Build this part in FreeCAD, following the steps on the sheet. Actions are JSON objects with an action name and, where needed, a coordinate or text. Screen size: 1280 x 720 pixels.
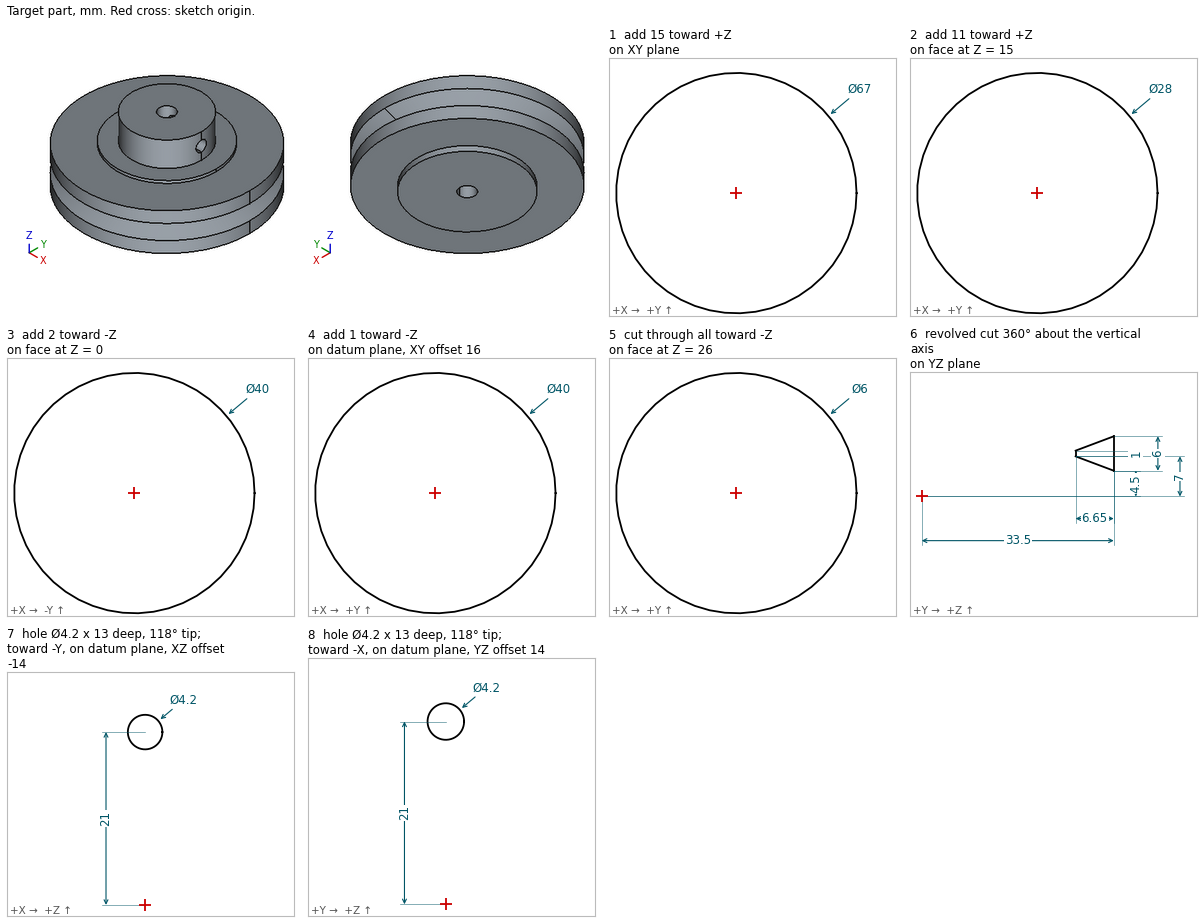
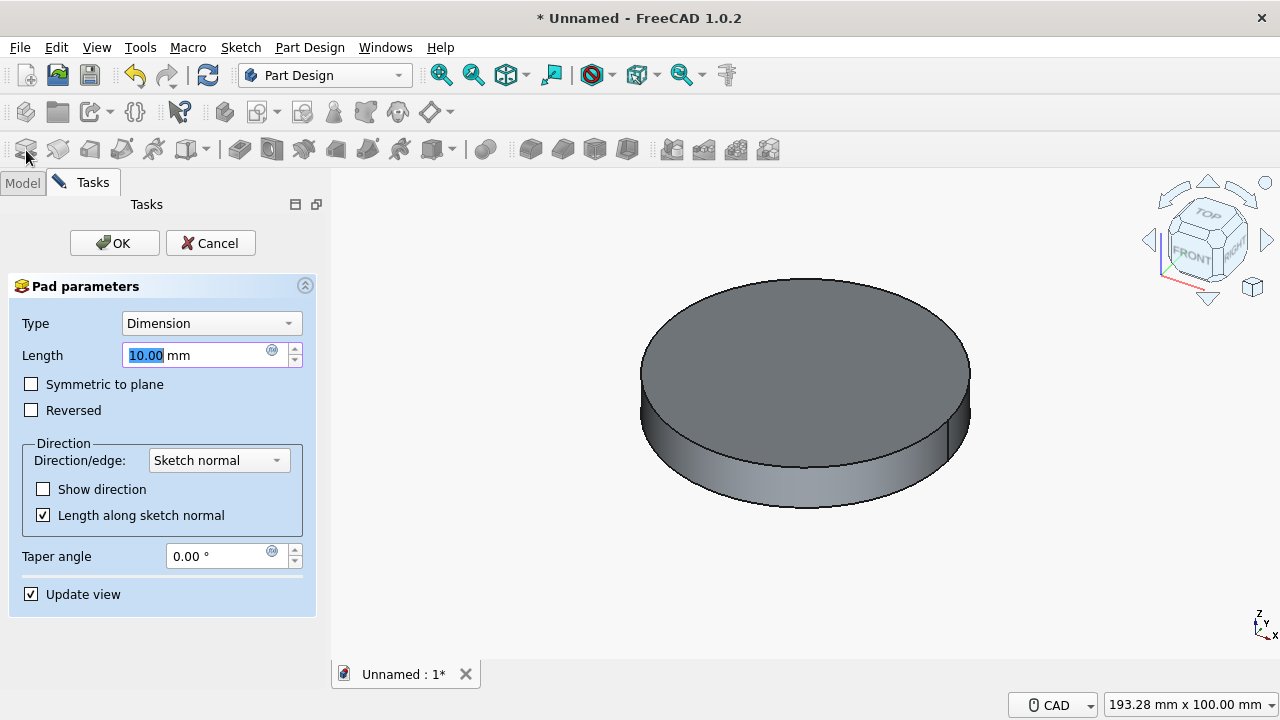
{"action": "type", "text": "15"}
{"action": "key", "text": "Tab"}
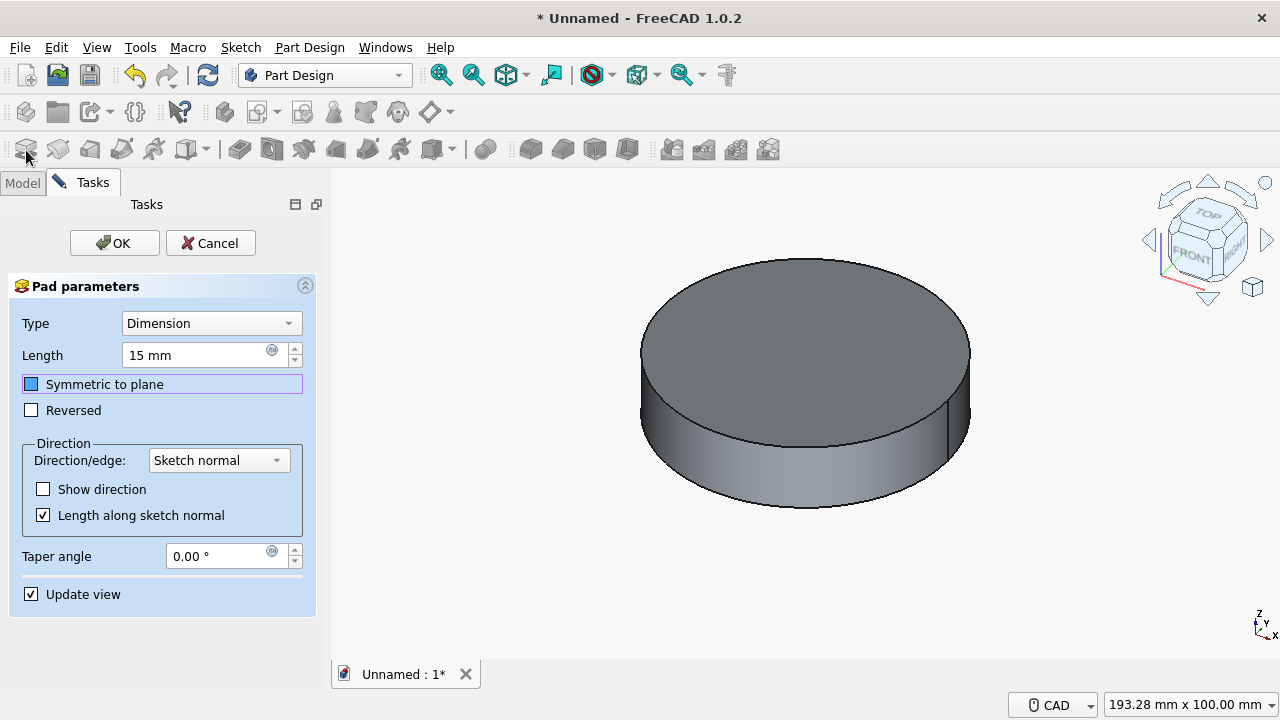
{"action": "left_click", "coordinate": [115, 243]}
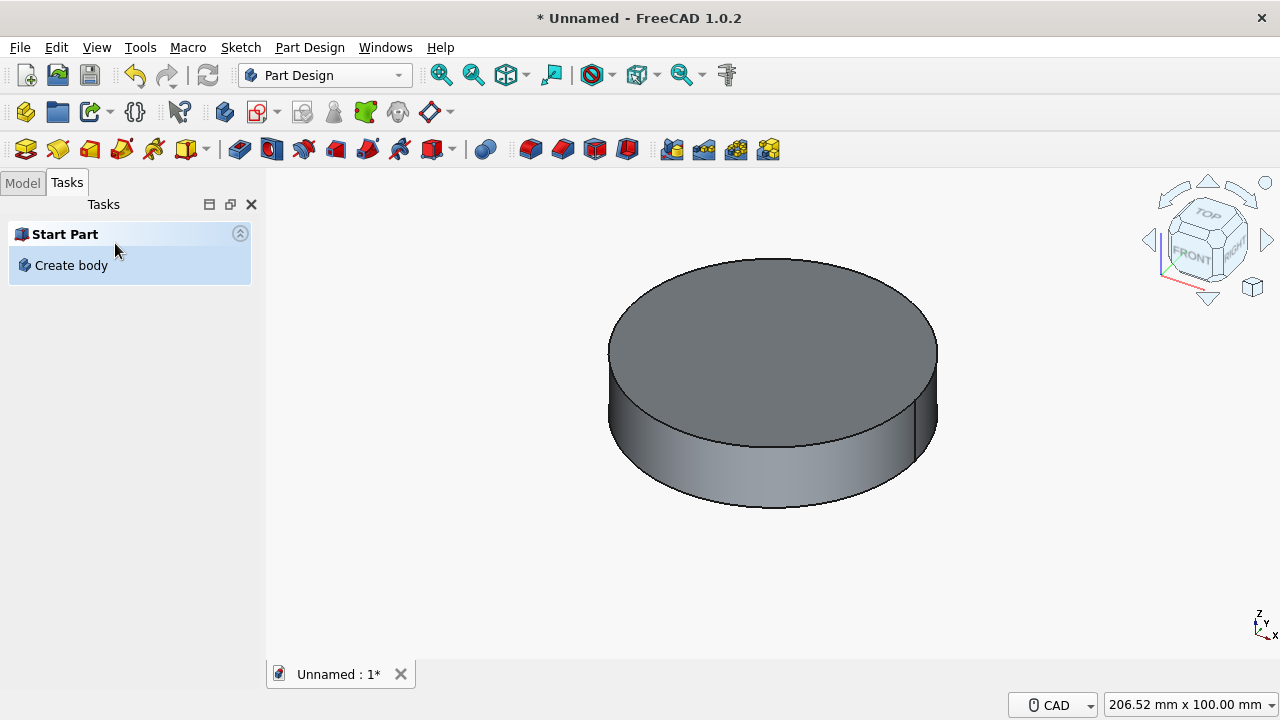
{"action": "left_click", "coordinate": [773, 352]}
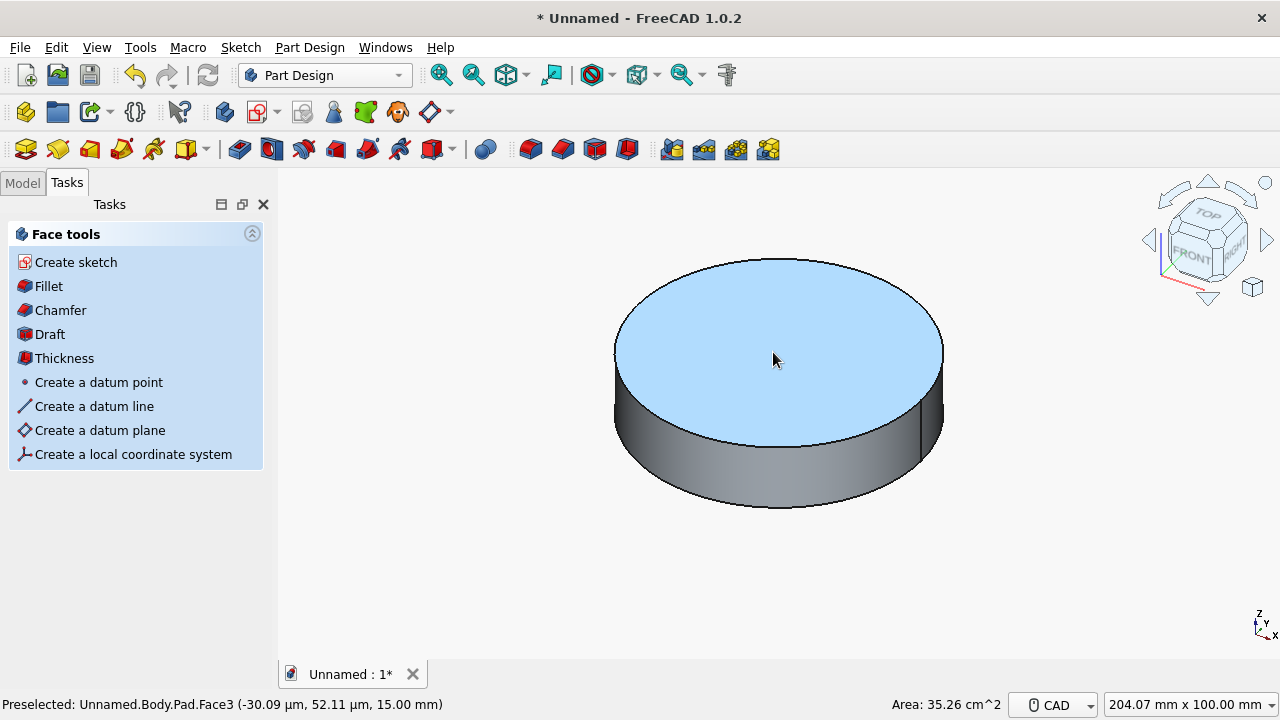
{"action": "left_click", "coordinate": [258, 112]}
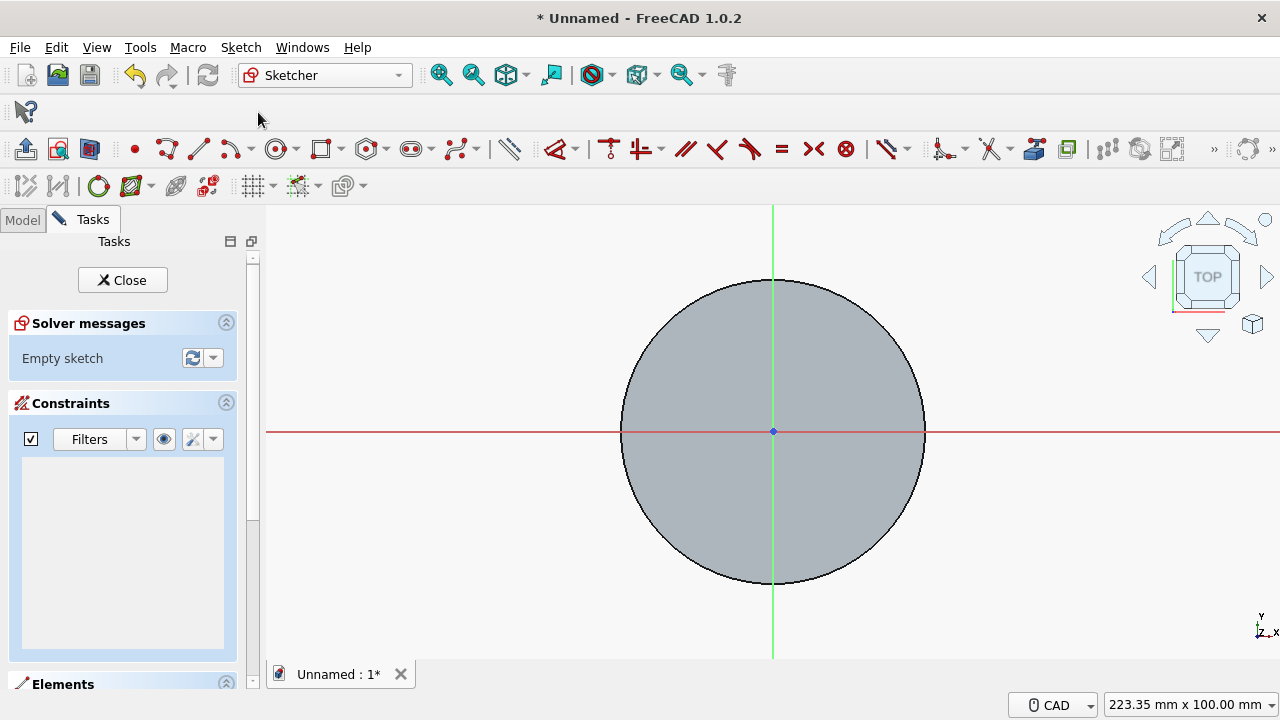
{"action": "scroll", "coordinate": [829, 432], "scroll_direction": "up", "scroll_amount": 4}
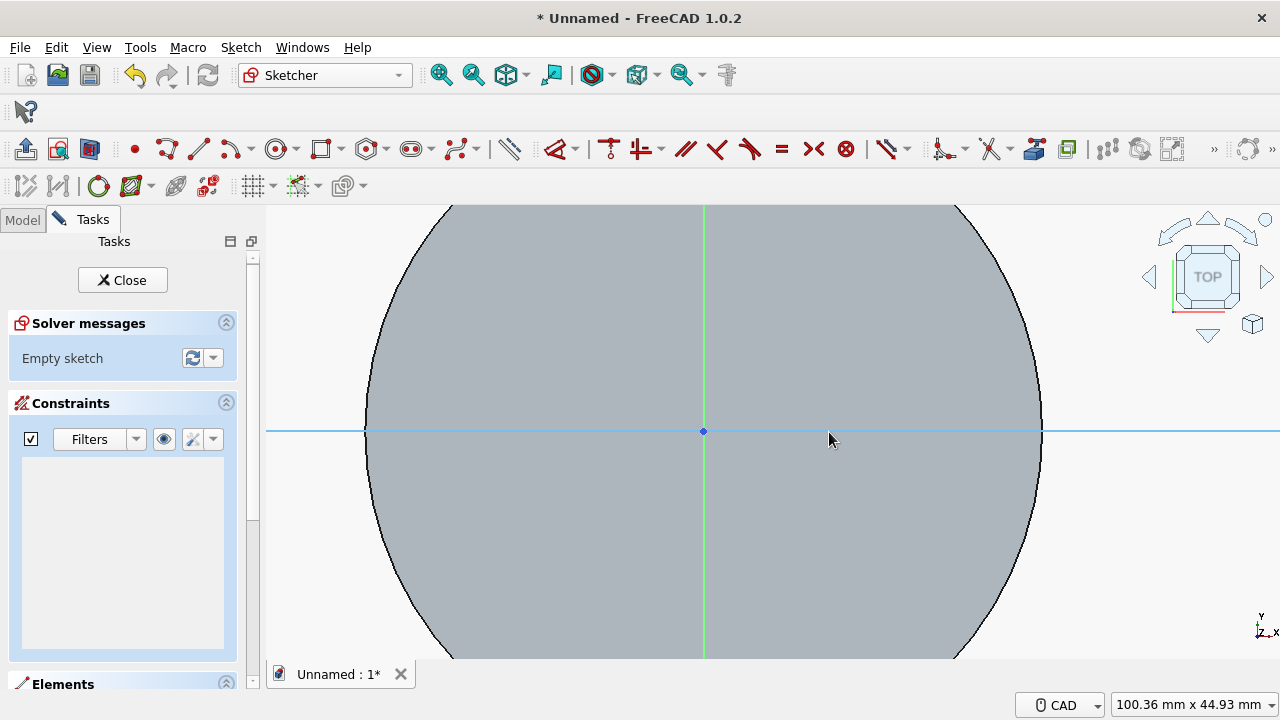
{"action": "key", "text": "g c"}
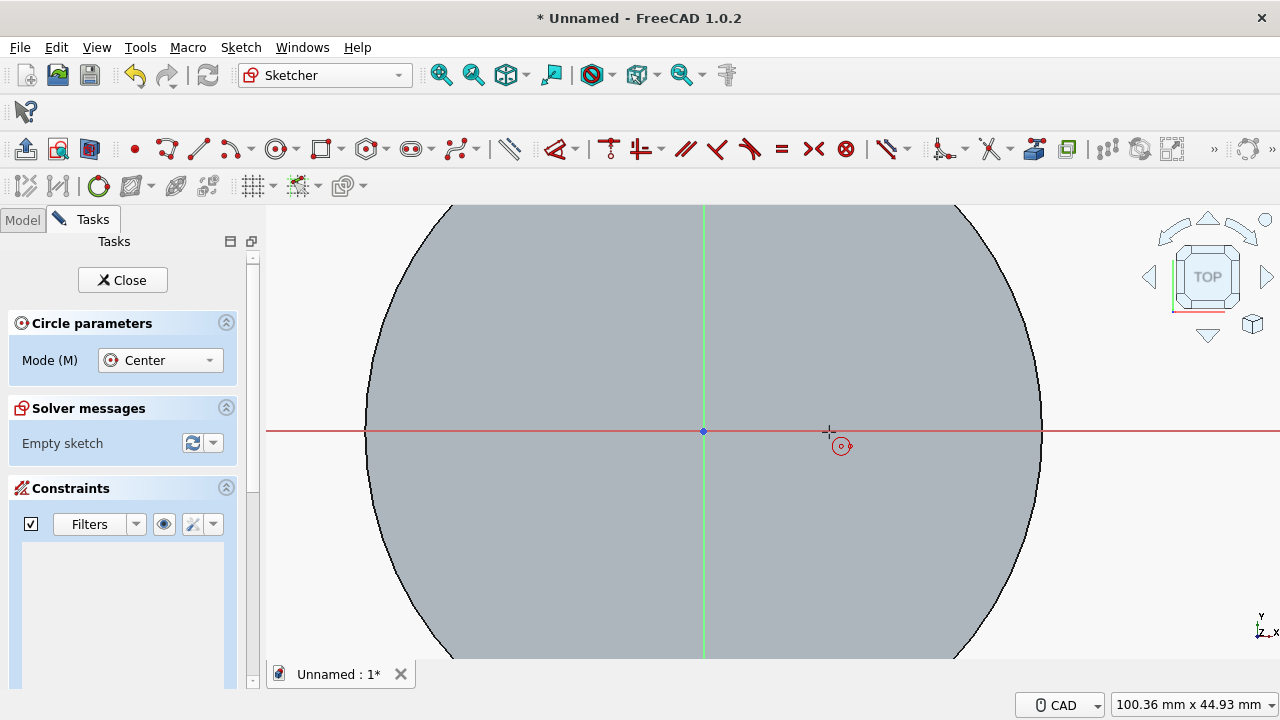
{"action": "left_click", "coordinate": [704, 431]}
{"action": "left_click", "coordinate": [804, 331]}
{"action": "key", "text": "Escape"}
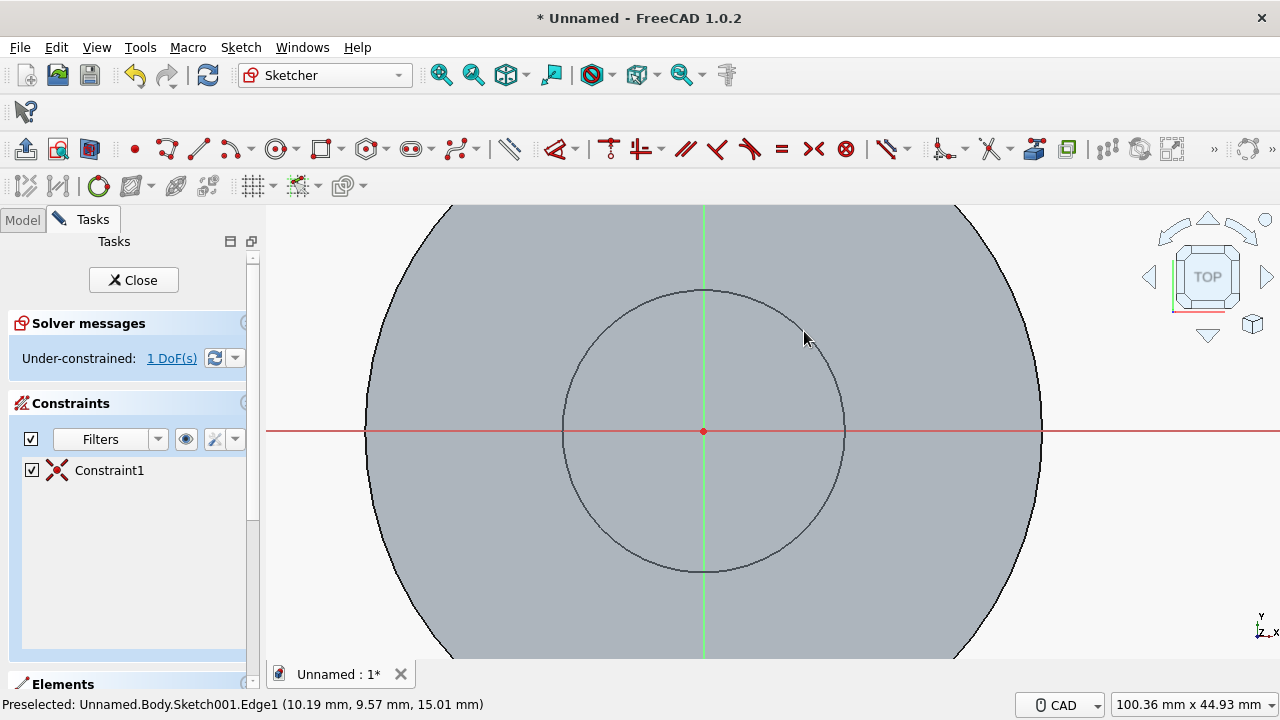
{"action": "left_click", "coordinate": [803, 331]}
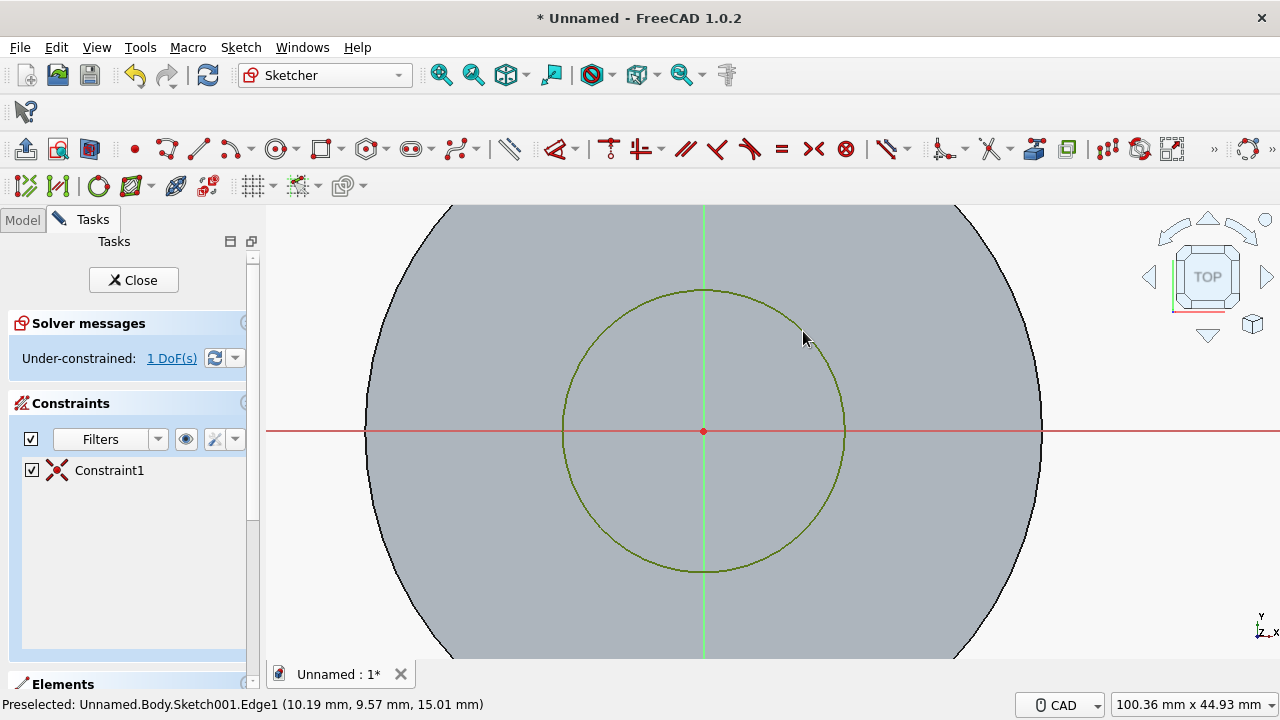
{"action": "left_click", "coordinate": [578, 150]}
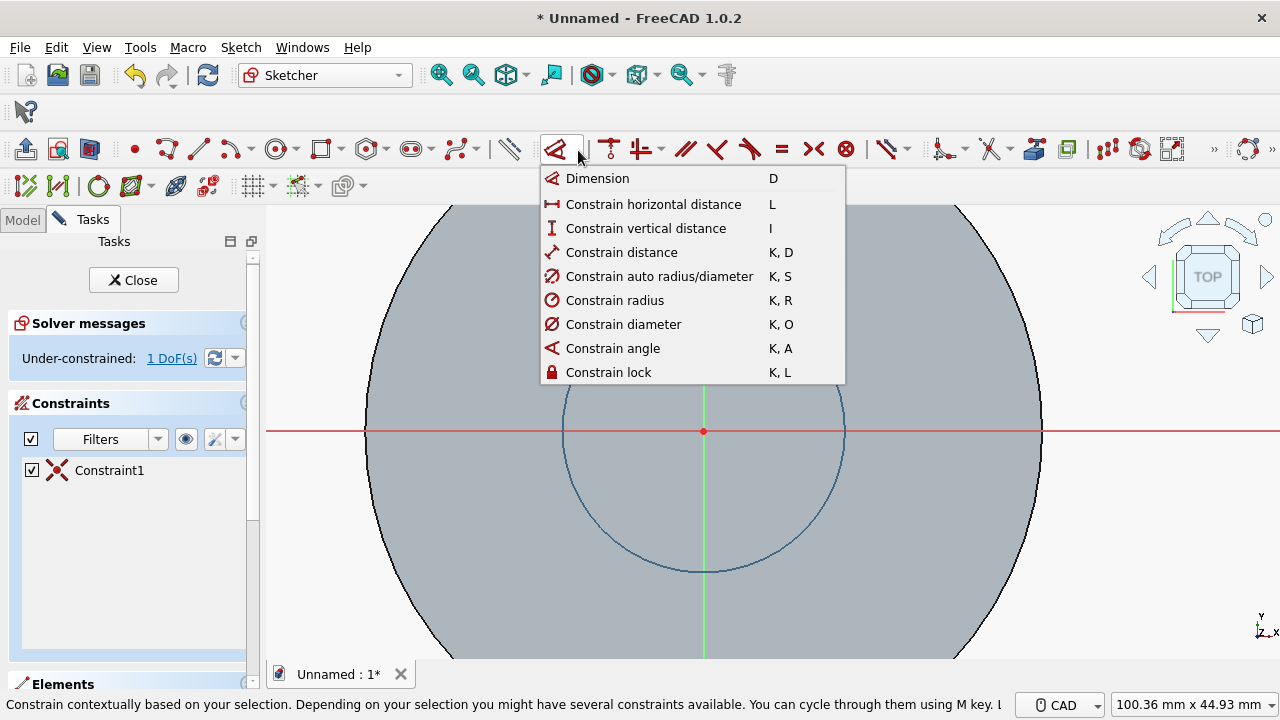
{"action": "left_click", "coordinate": [693, 324]}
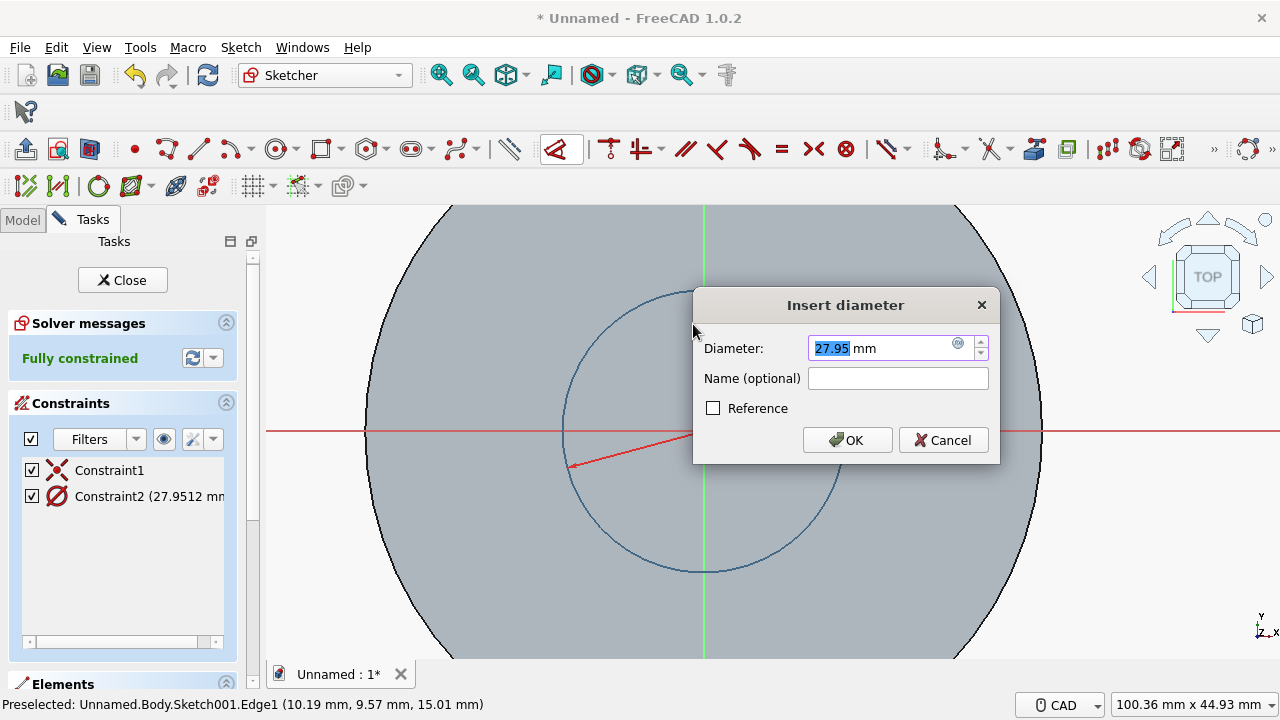
{"action": "type", "text": "28"}
{"action": "key", "text": "Return"}